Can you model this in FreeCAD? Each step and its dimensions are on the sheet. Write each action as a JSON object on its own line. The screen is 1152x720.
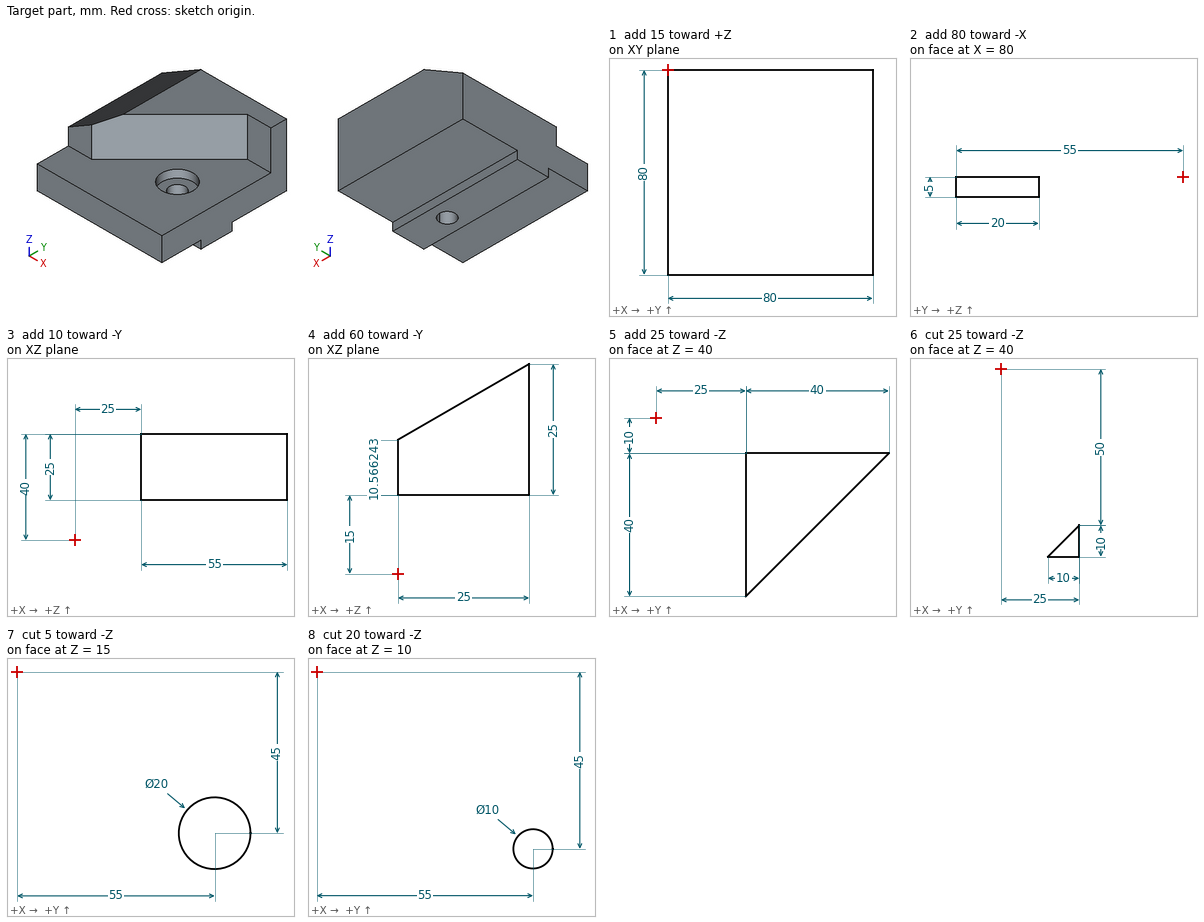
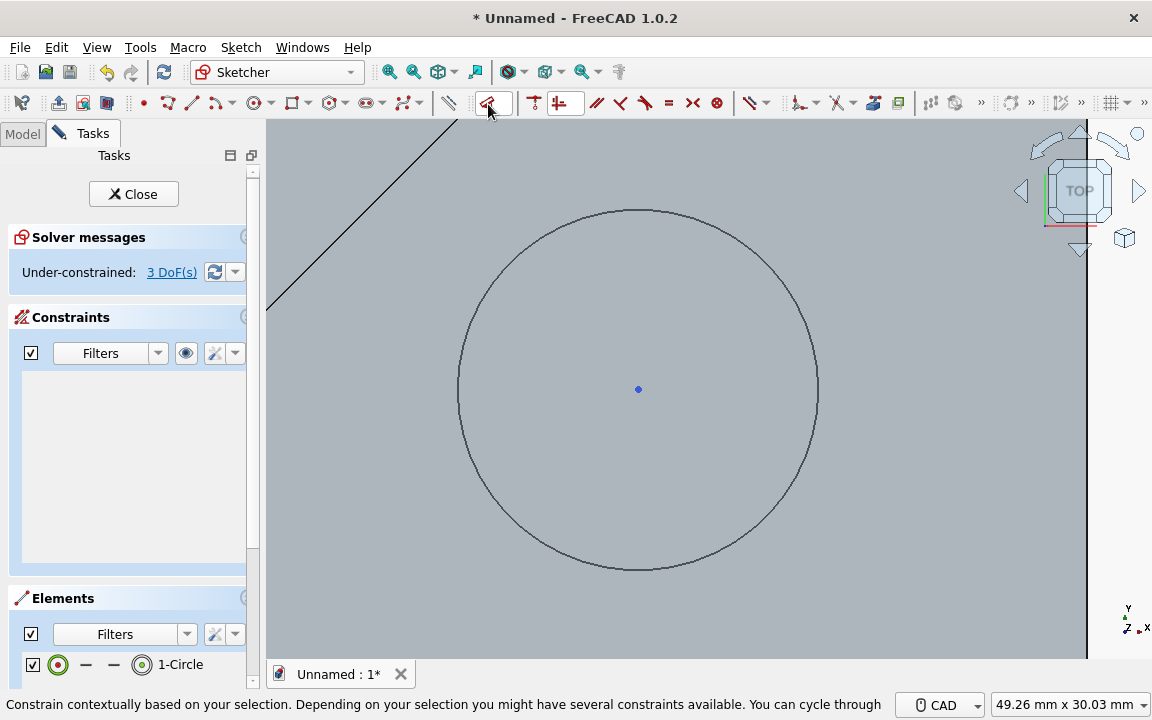
{"action": "left_click", "coordinate": [765, 262]}
{"action": "left_click", "coordinate": [788, 239]}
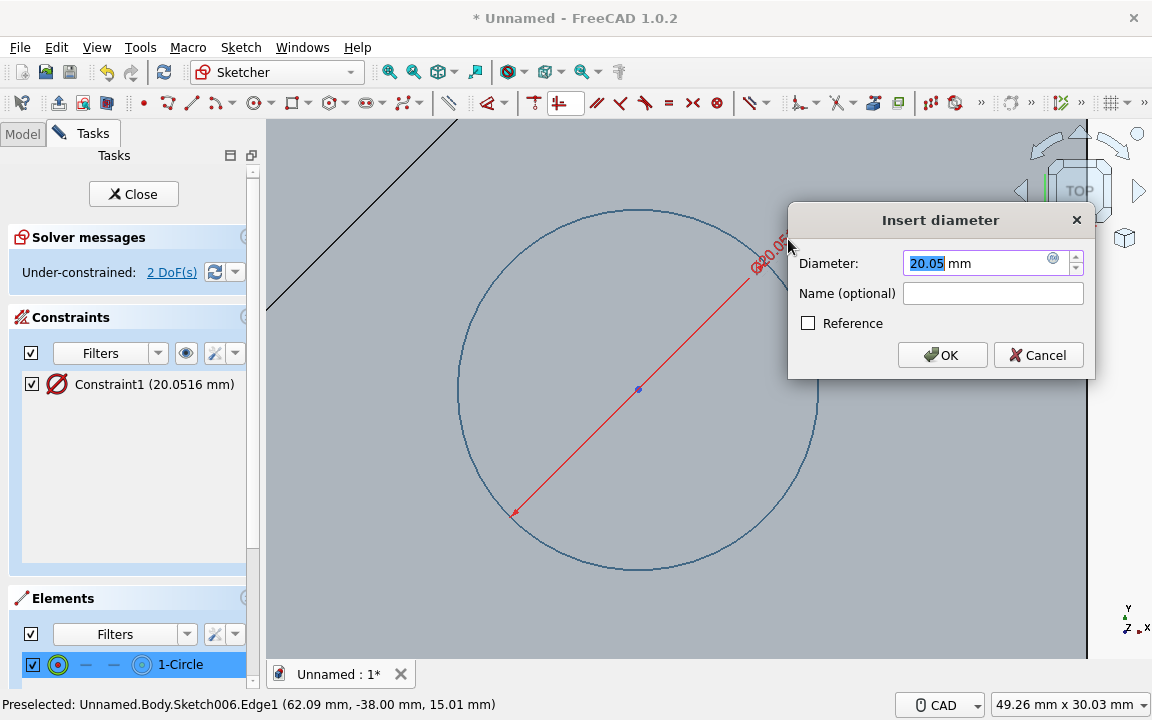
{"action": "type", "text": "20"}
{"action": "key", "text": "Return"}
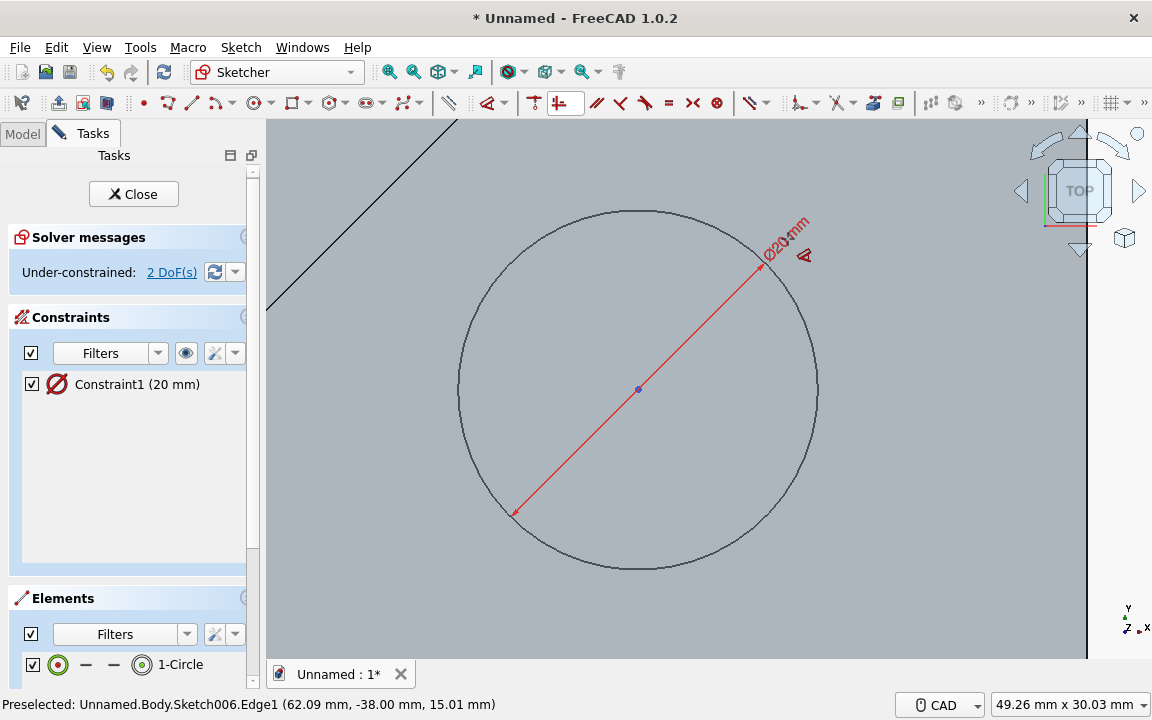
{"action": "left_click", "coordinate": [638, 390]}
{"action": "left_click", "coordinate": [387, 424]}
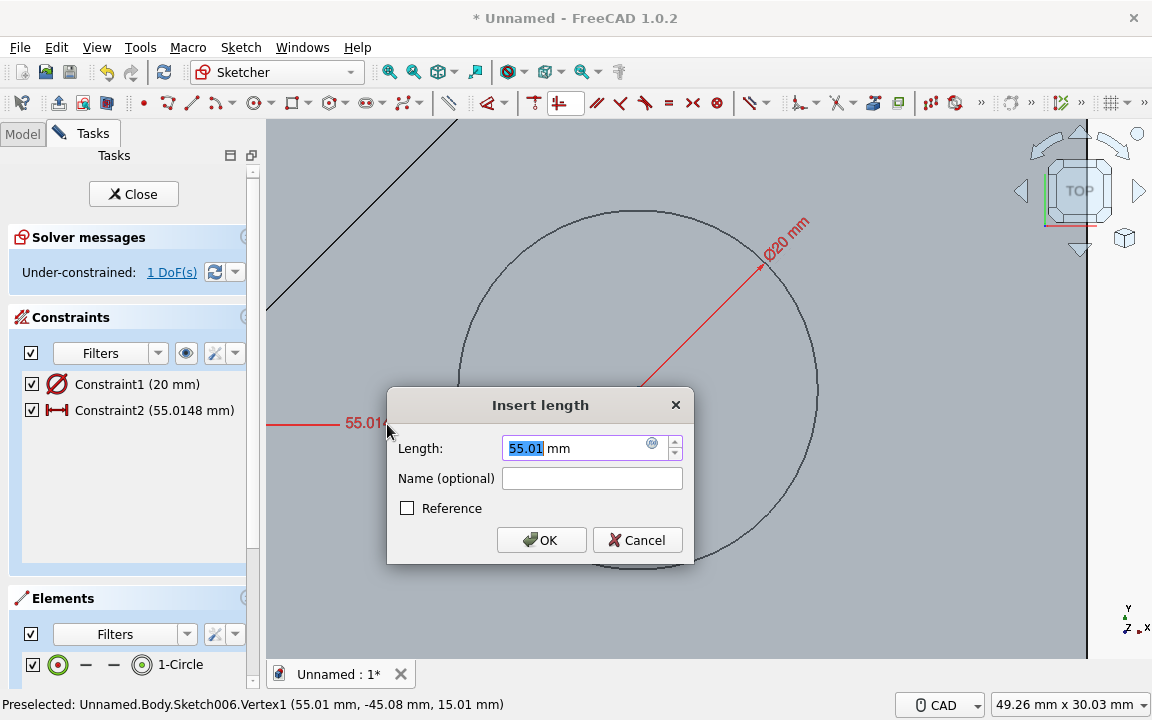
{"action": "type", "text": "55"}
{"action": "key", "text": "Return"}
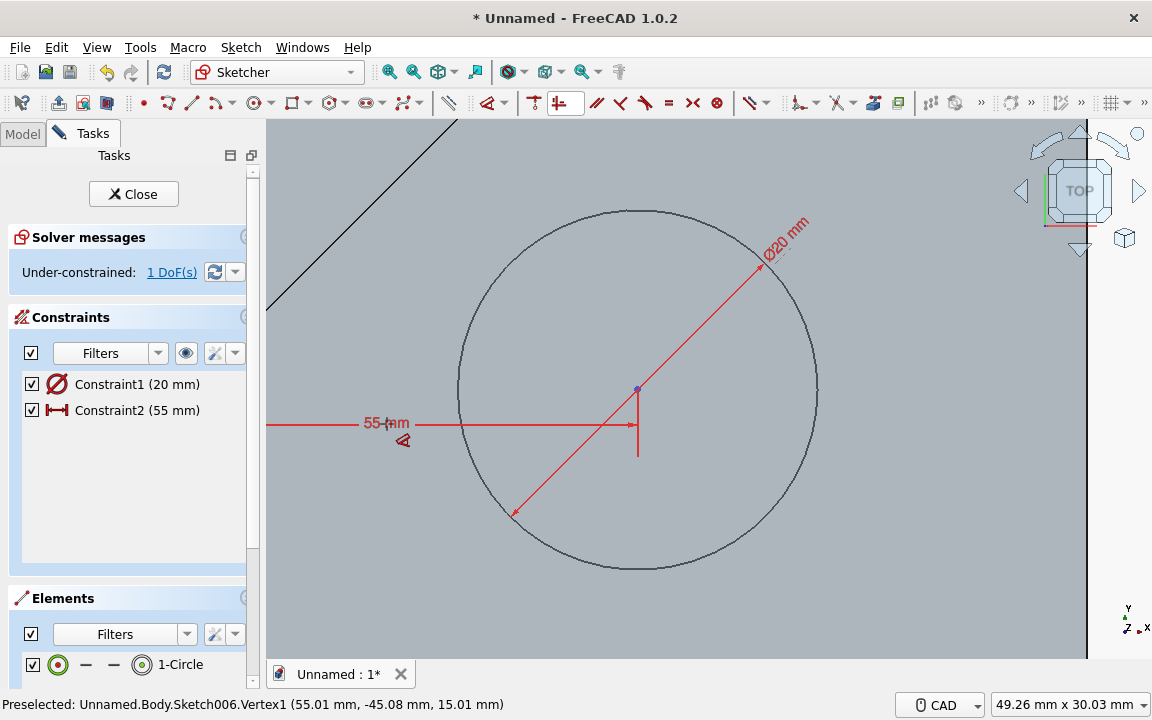
{"action": "left_click", "coordinate": [638, 390]}
{"action": "left_click", "coordinate": [672, 269]}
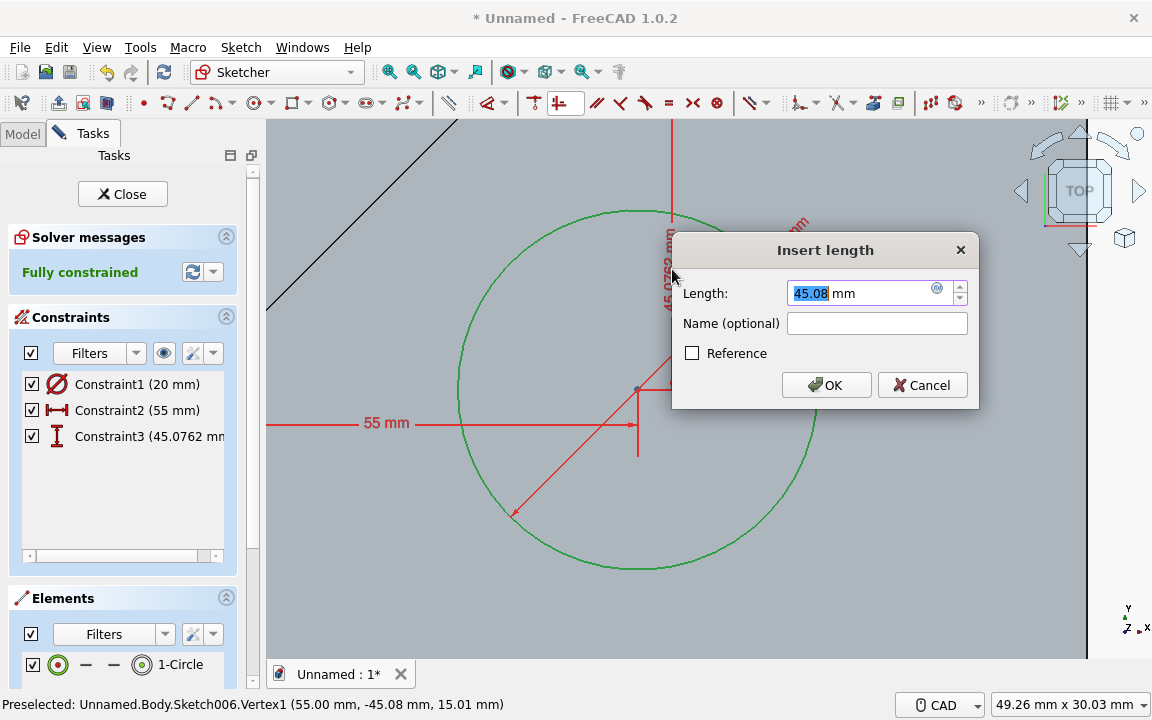
{"action": "type", "text": "45"}
{"action": "key", "text": "Return"}
{"action": "key", "text": "Escape"}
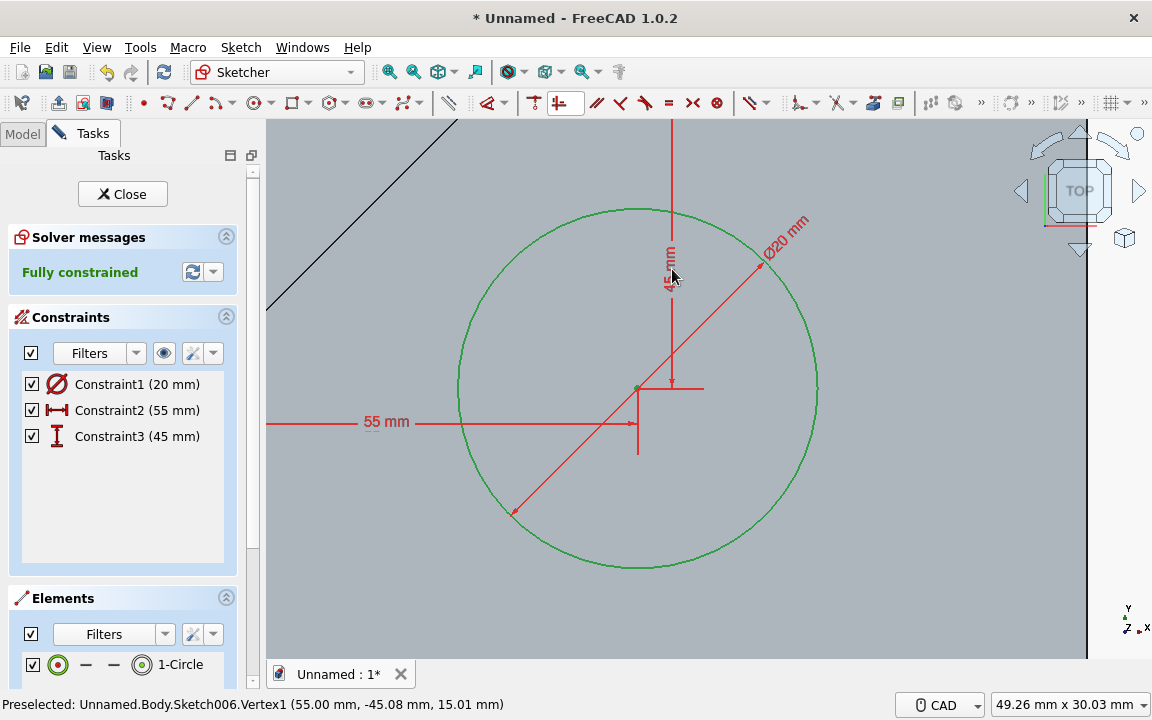
{"action": "left_click", "coordinate": [123, 194]}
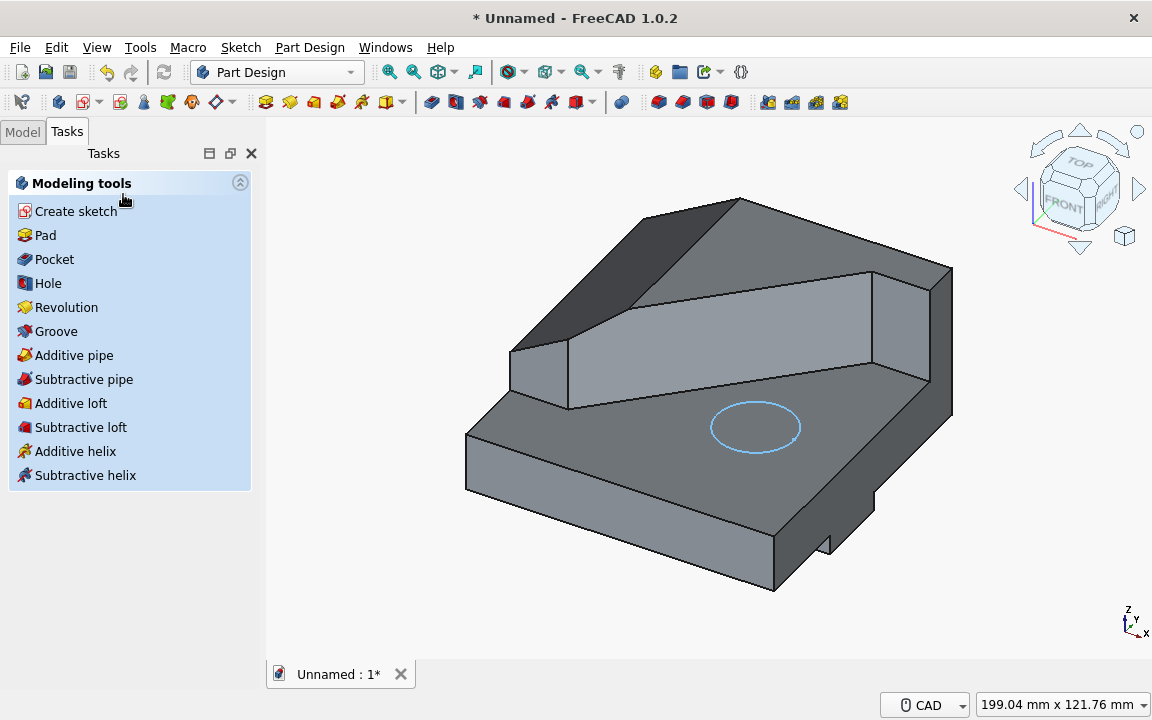
{"action": "left_click", "coordinate": [432, 102]}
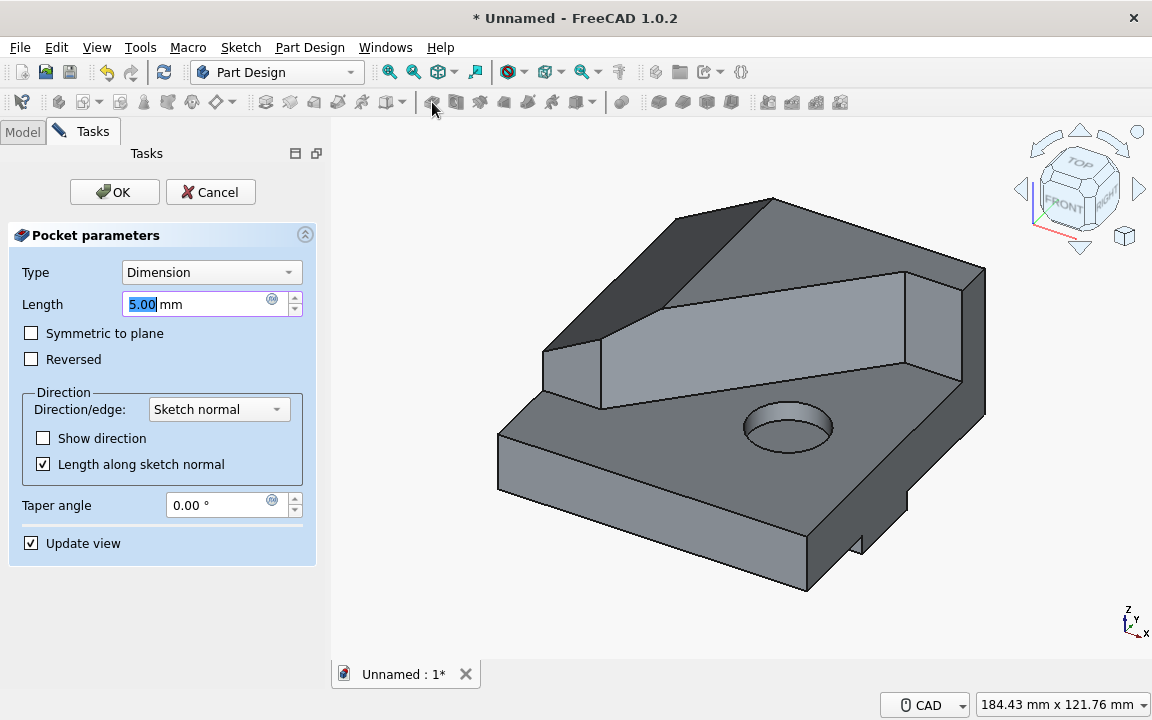
{"action": "type", "text": "5"}
{"action": "key", "text": "Tab"}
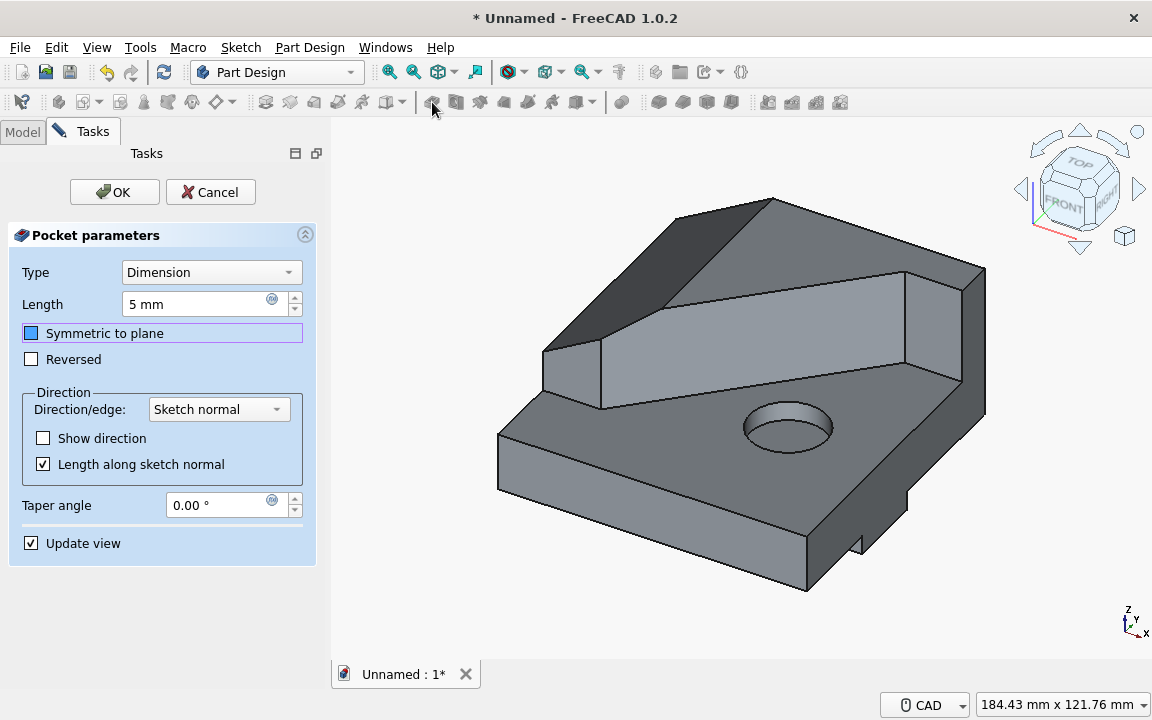
{"action": "left_click", "coordinate": [115, 192]}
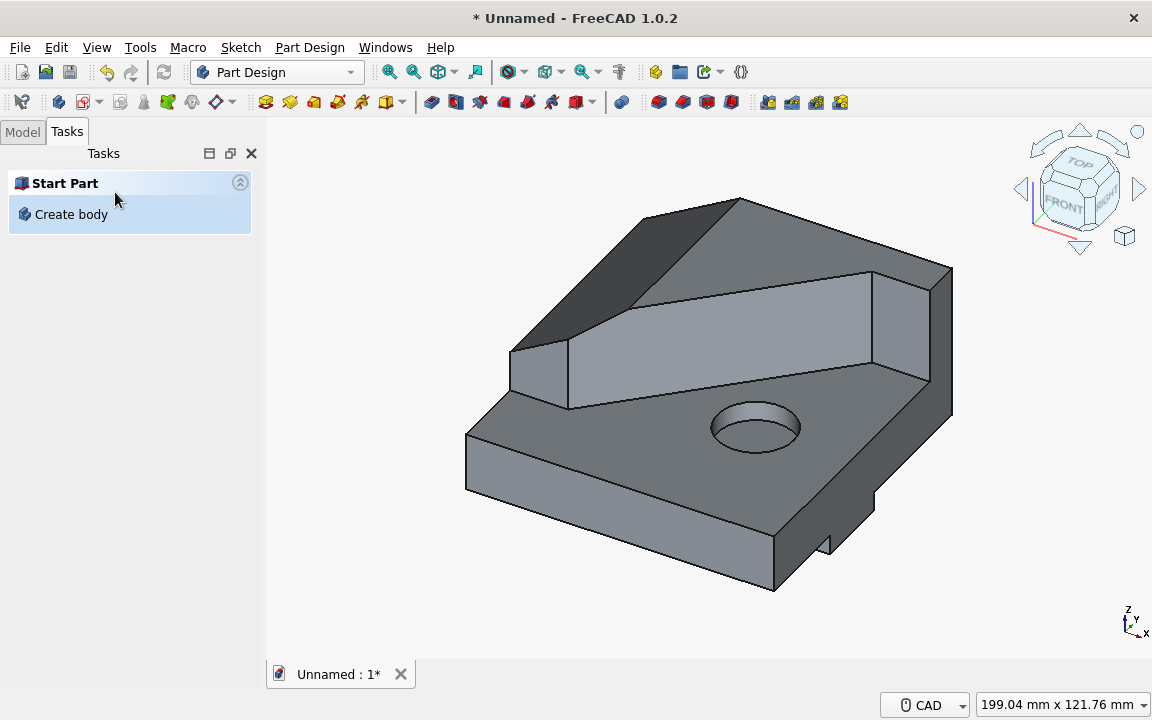
{"action": "left_click", "coordinate": [745, 441]}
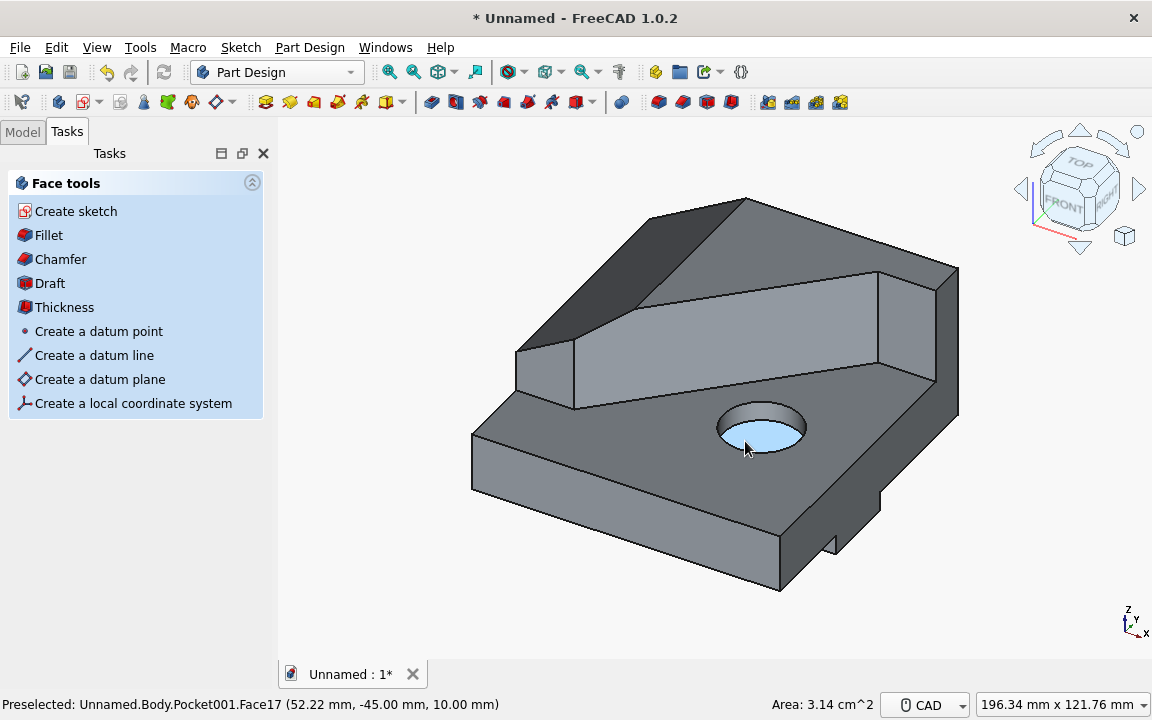
{"action": "left_click", "coordinate": [84, 102]}